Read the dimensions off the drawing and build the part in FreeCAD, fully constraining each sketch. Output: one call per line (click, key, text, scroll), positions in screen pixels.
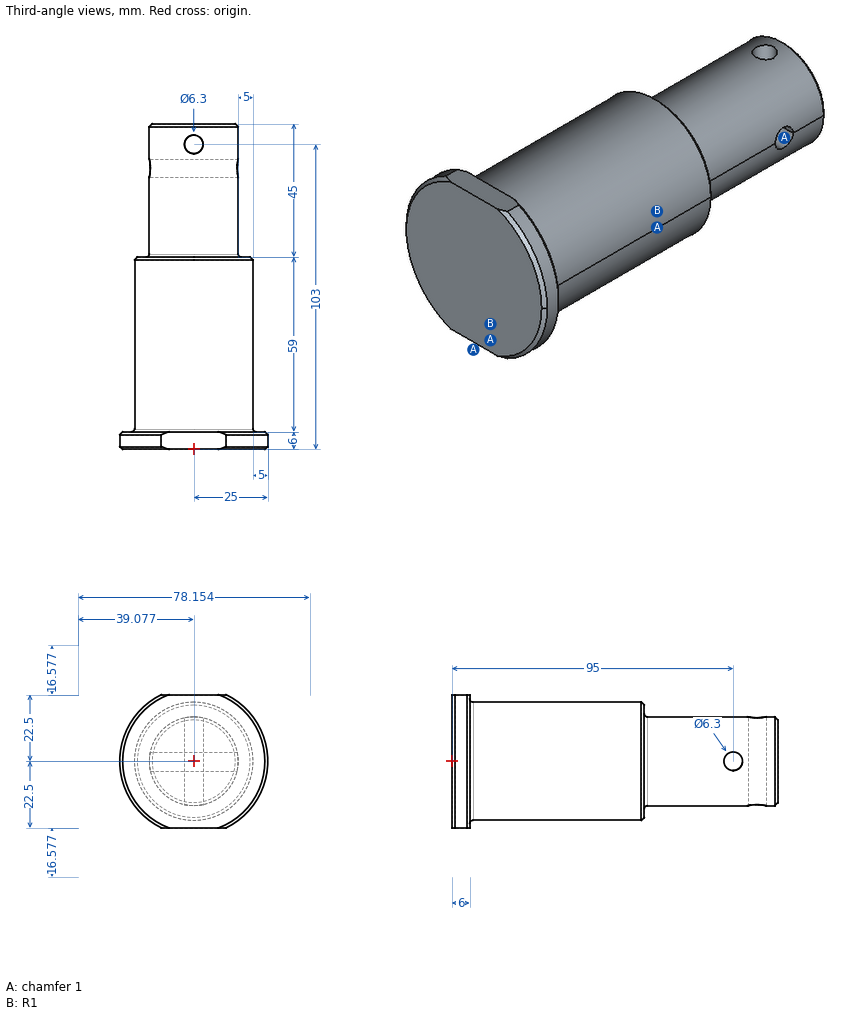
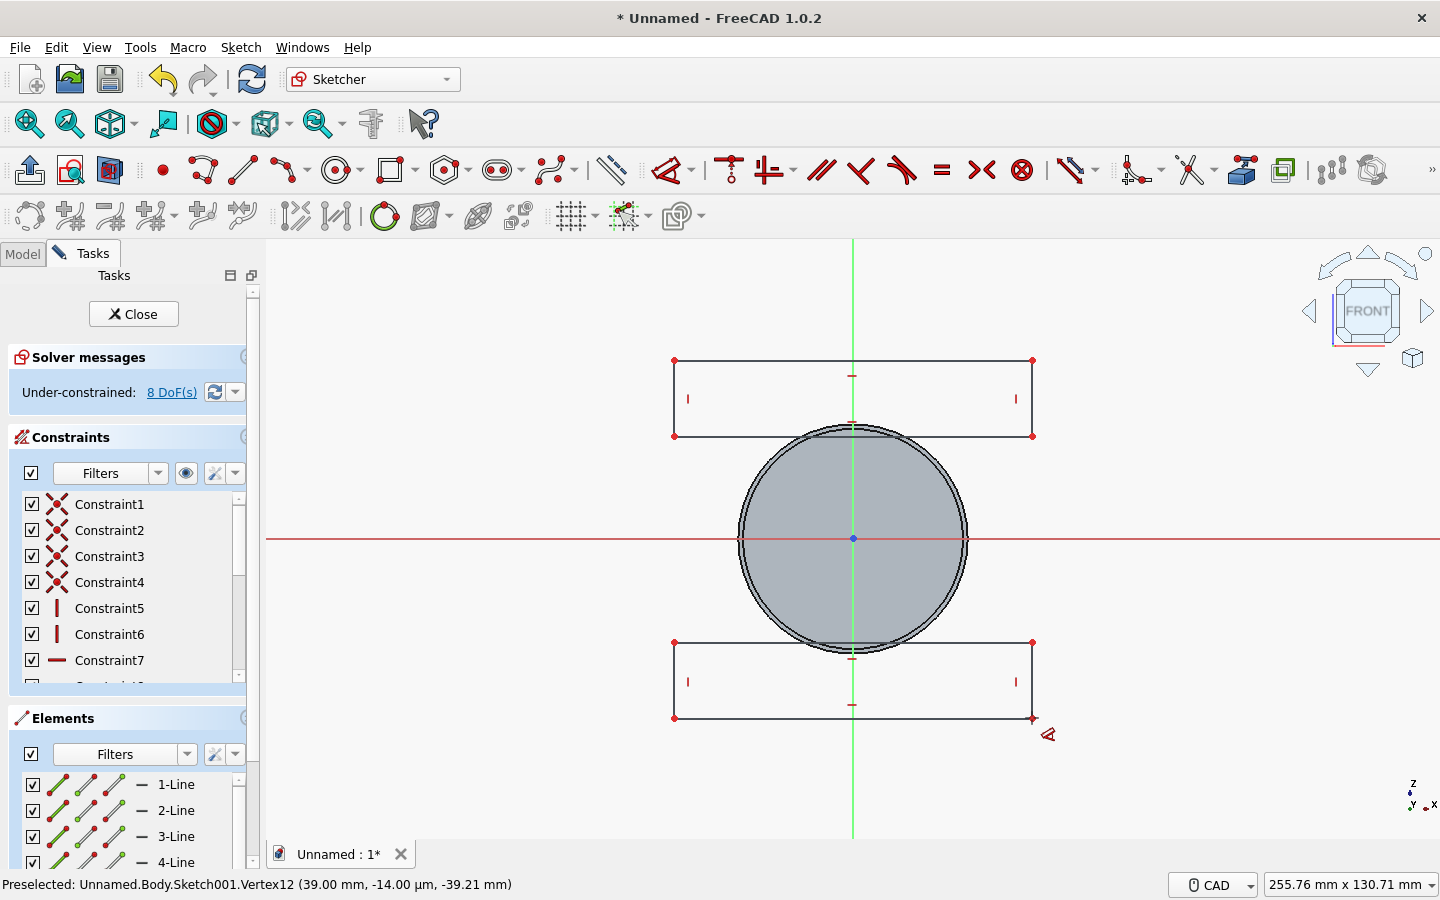
click(674, 437)
click(640, 488)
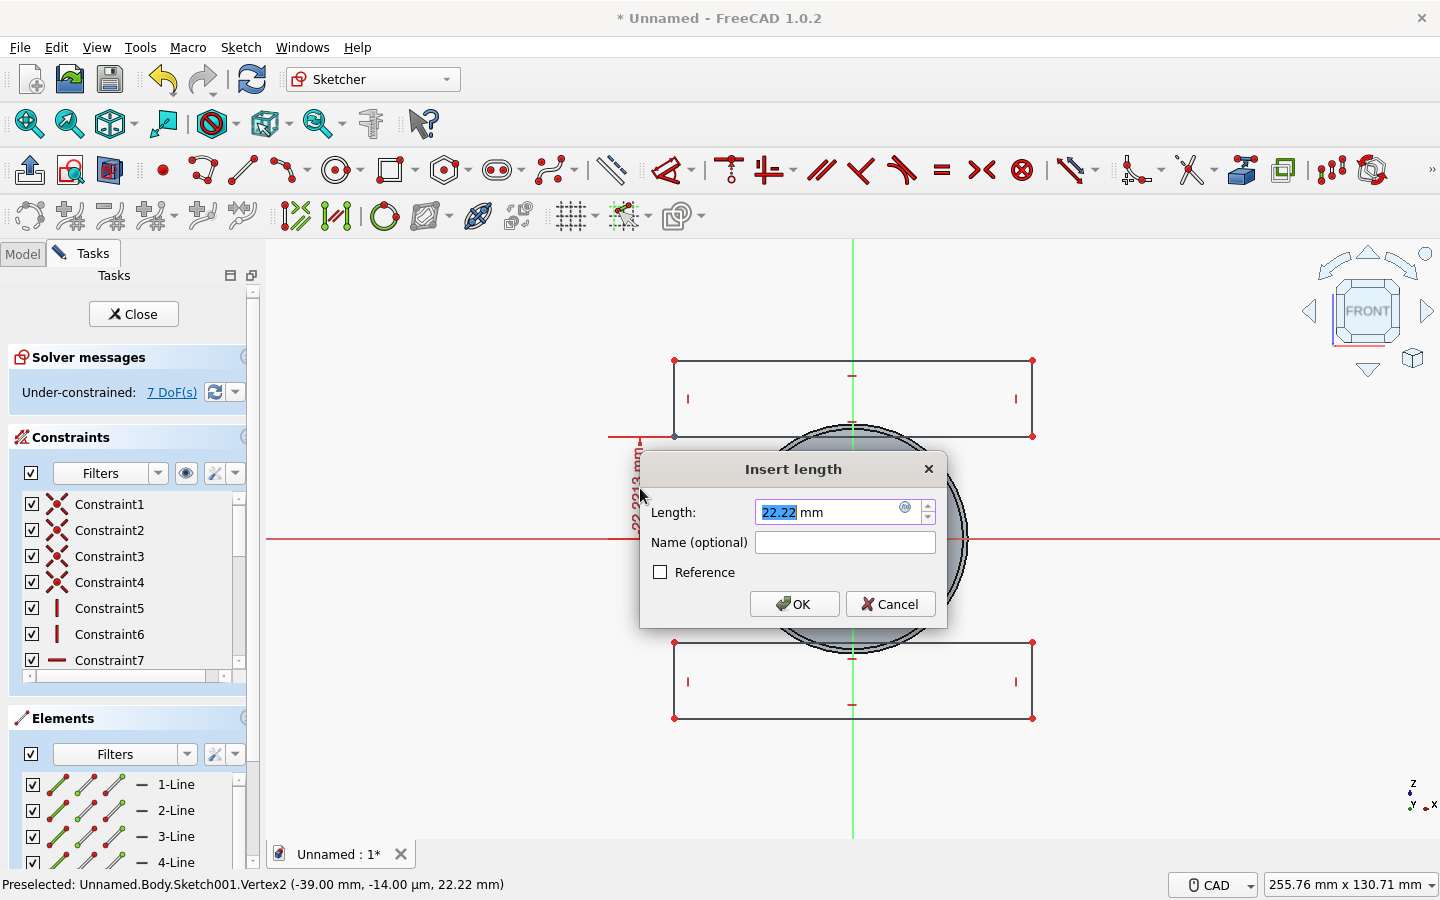
text(22.5)
key(Return)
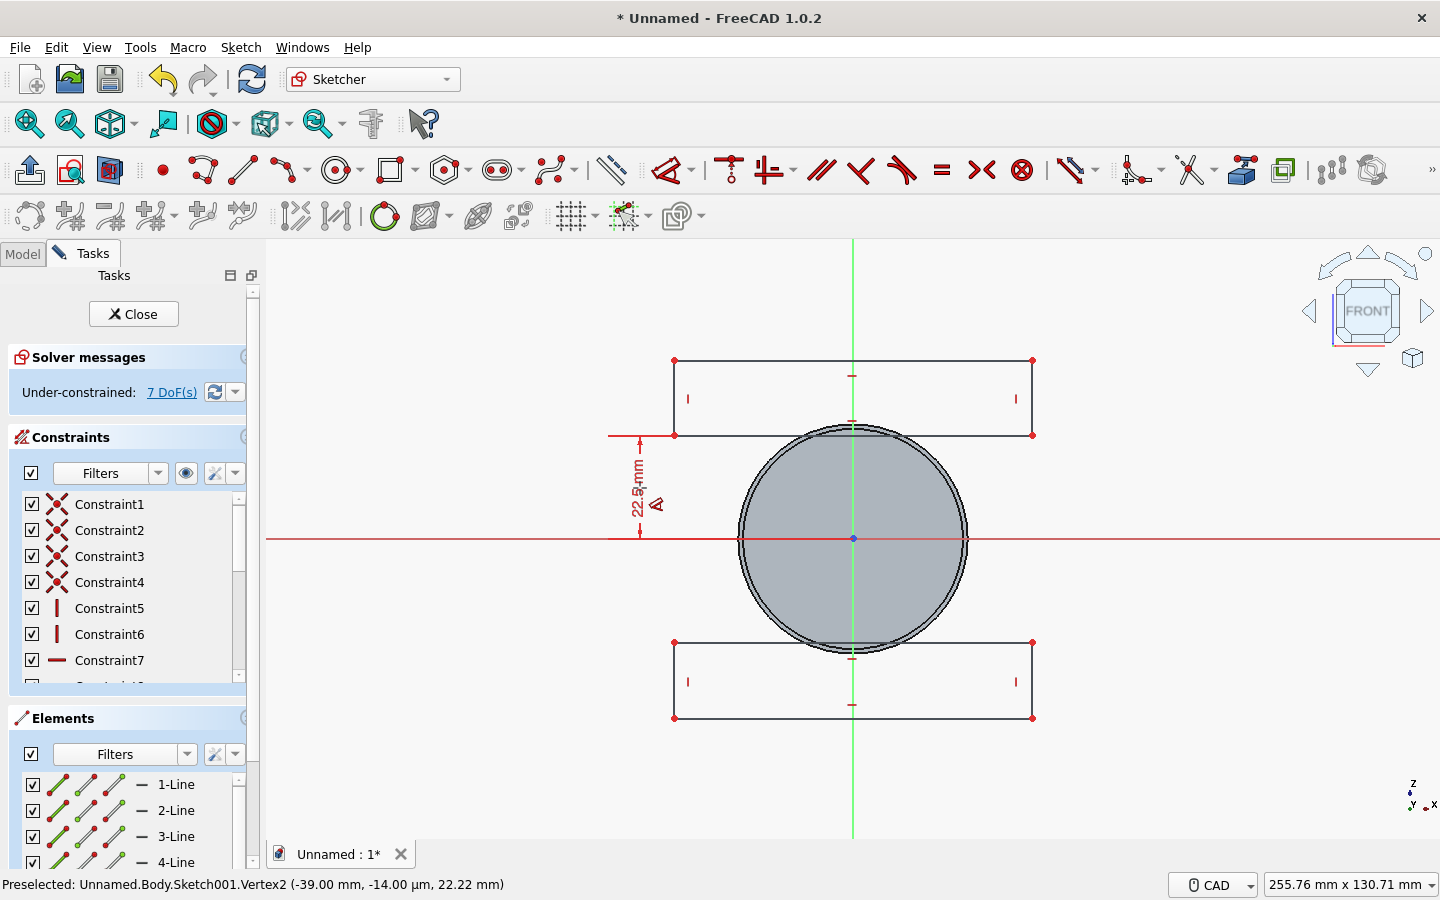
click(674, 643)
click(640, 591)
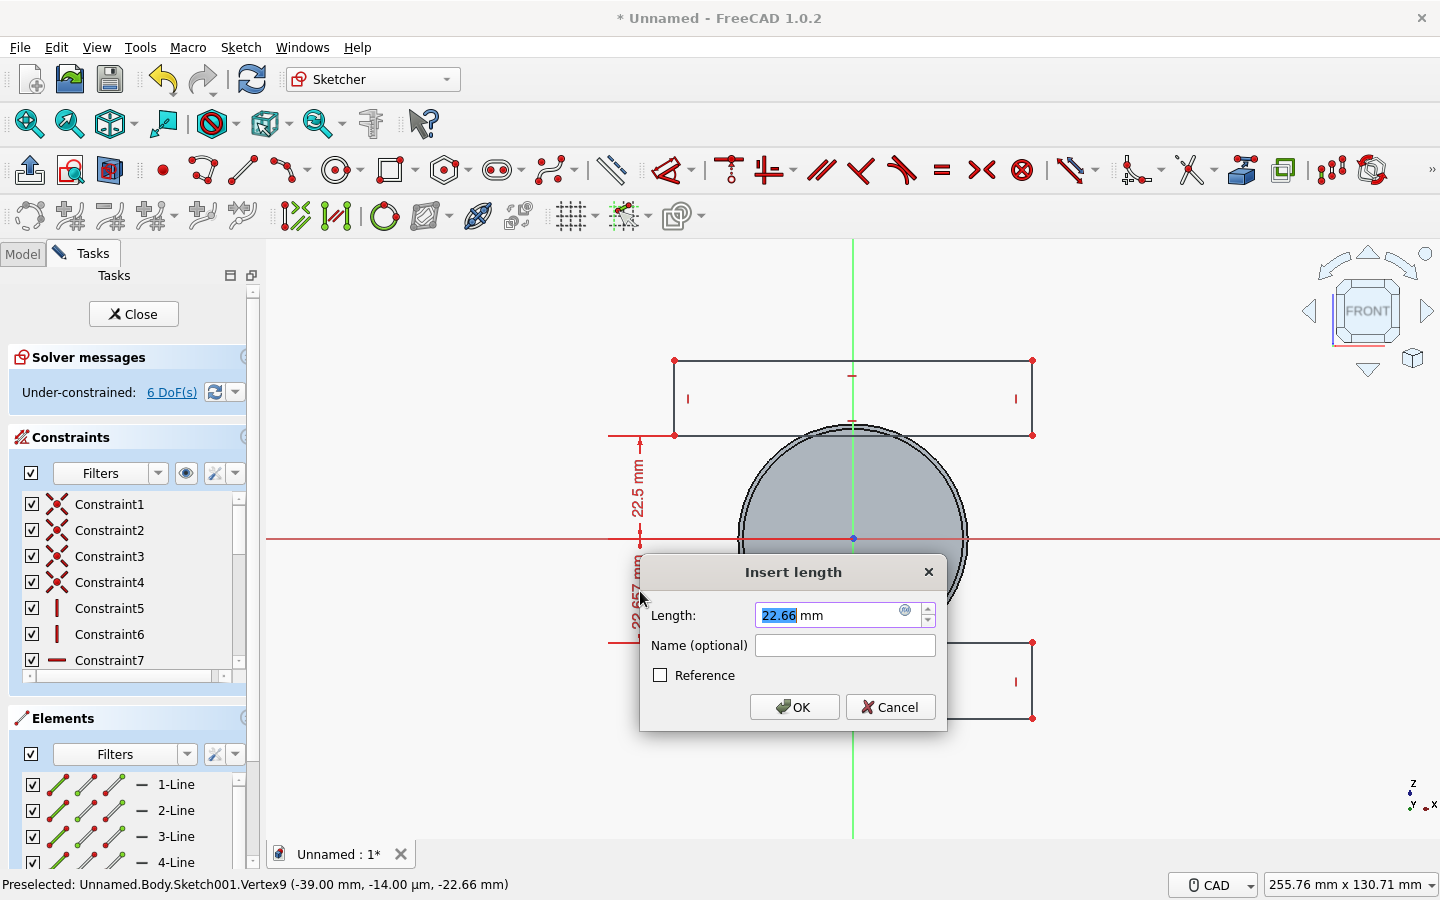
text(22.5)
key(Return)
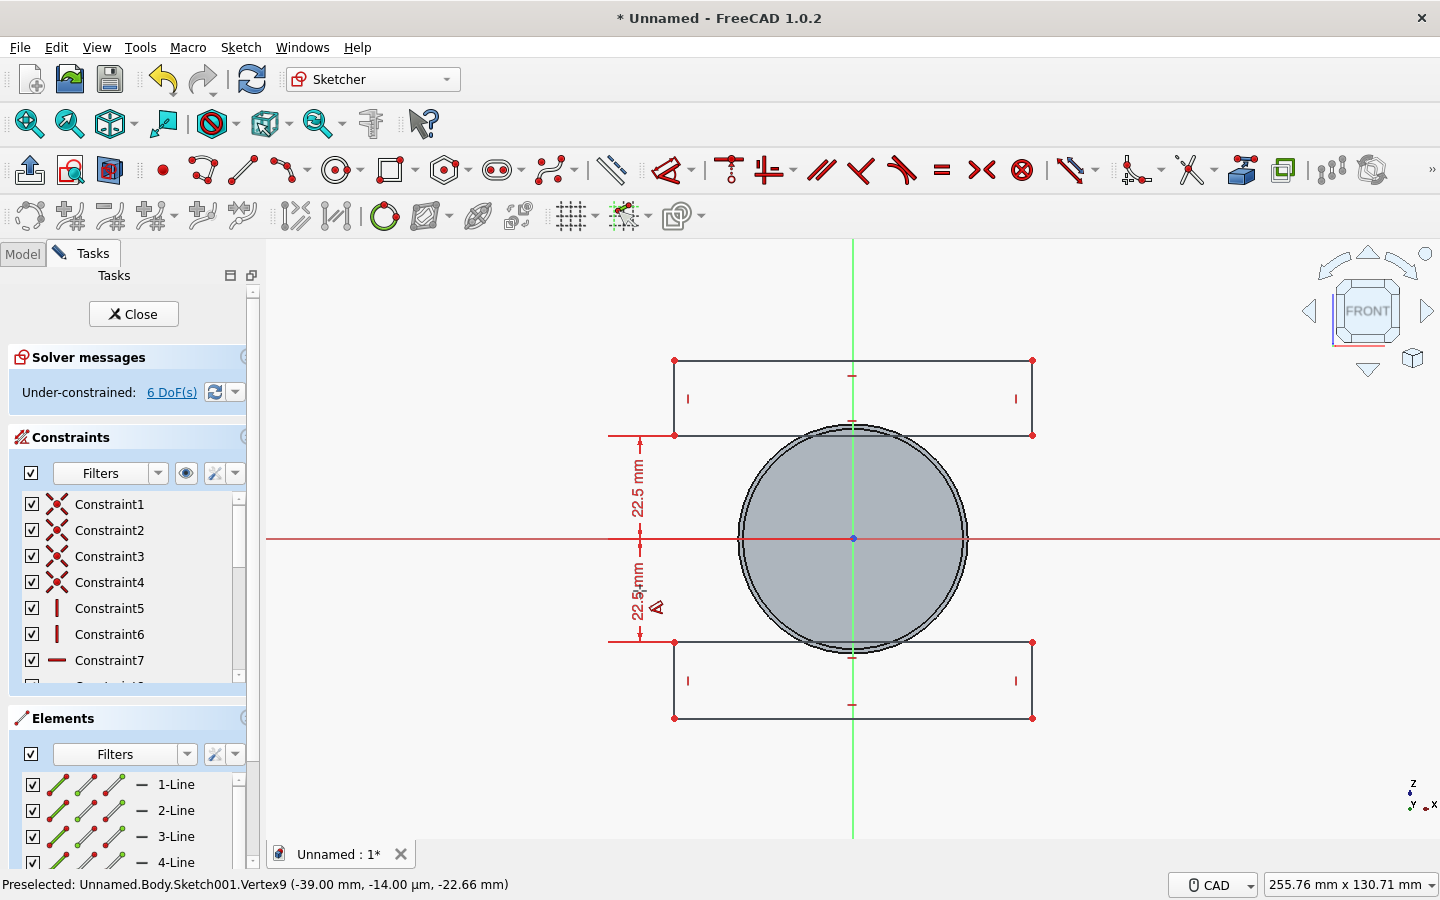
click(674, 383)
click(640, 398)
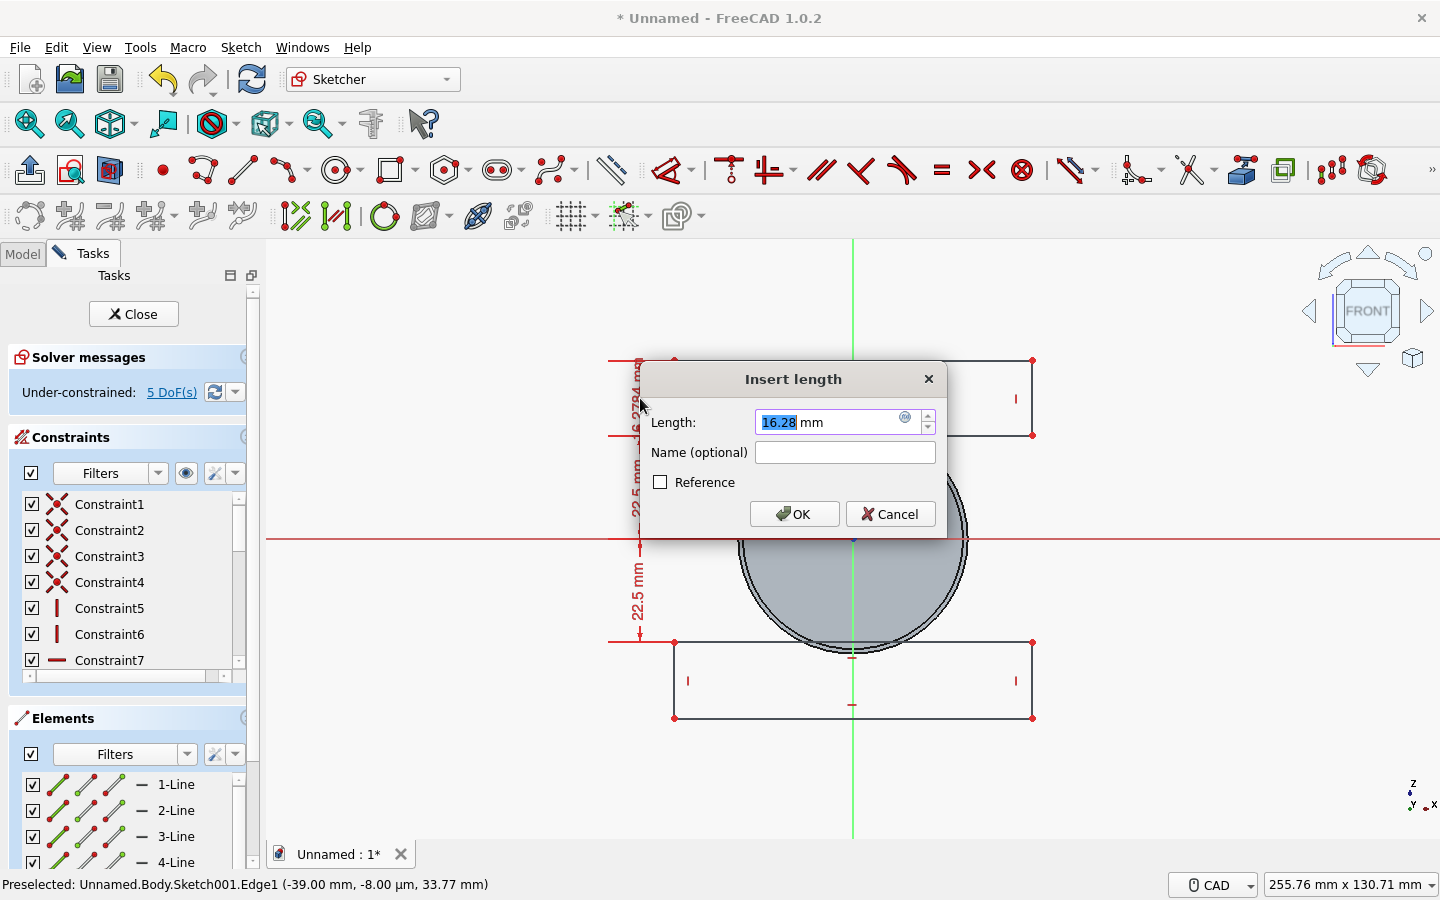
text(16.577)
key(Return)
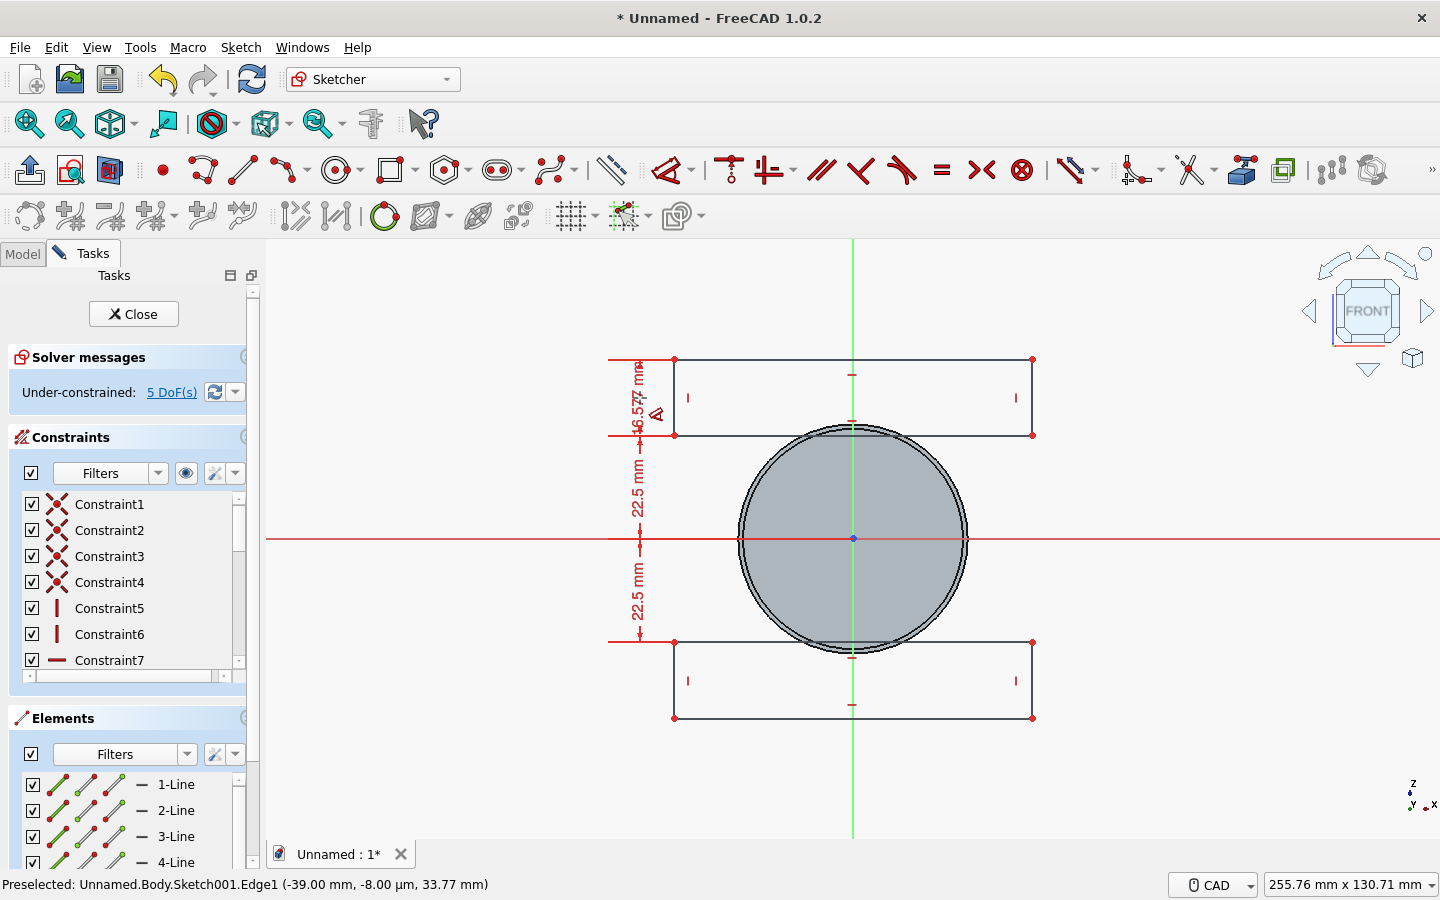
click(781, 436)
click(771, 402)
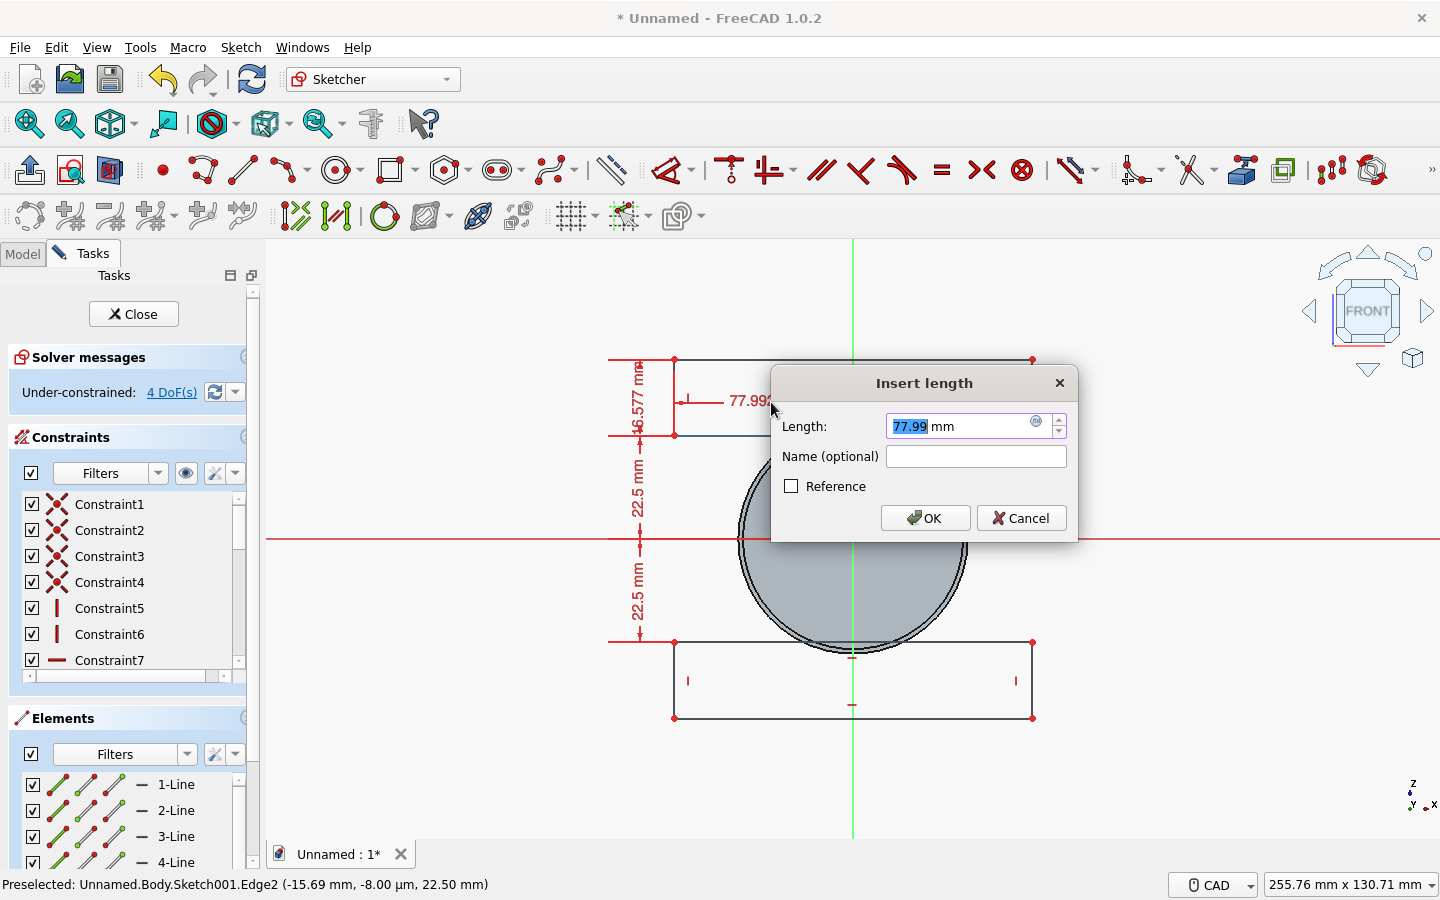
text(78.154)
key(Return)